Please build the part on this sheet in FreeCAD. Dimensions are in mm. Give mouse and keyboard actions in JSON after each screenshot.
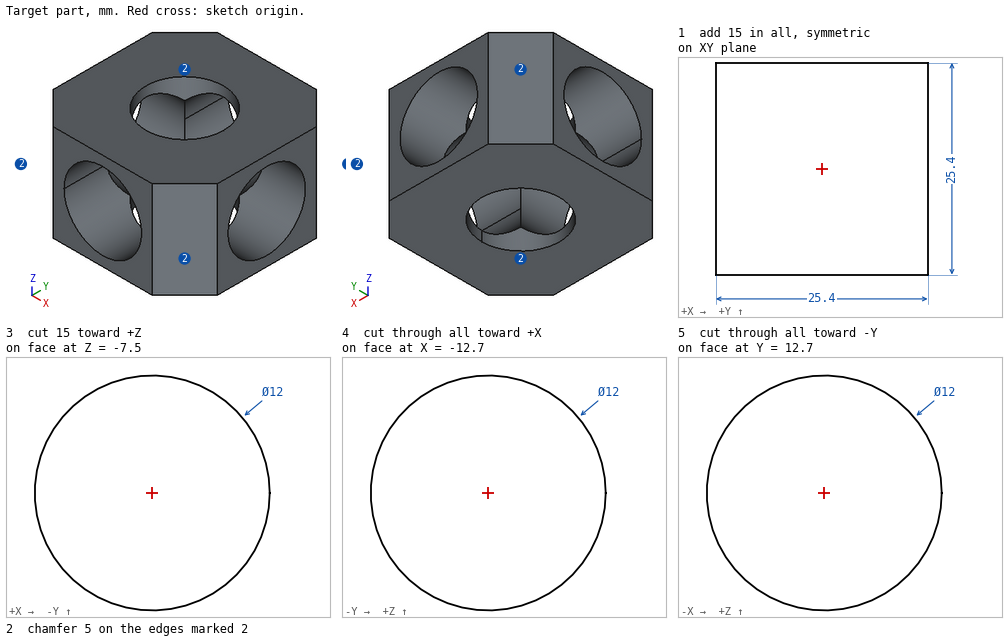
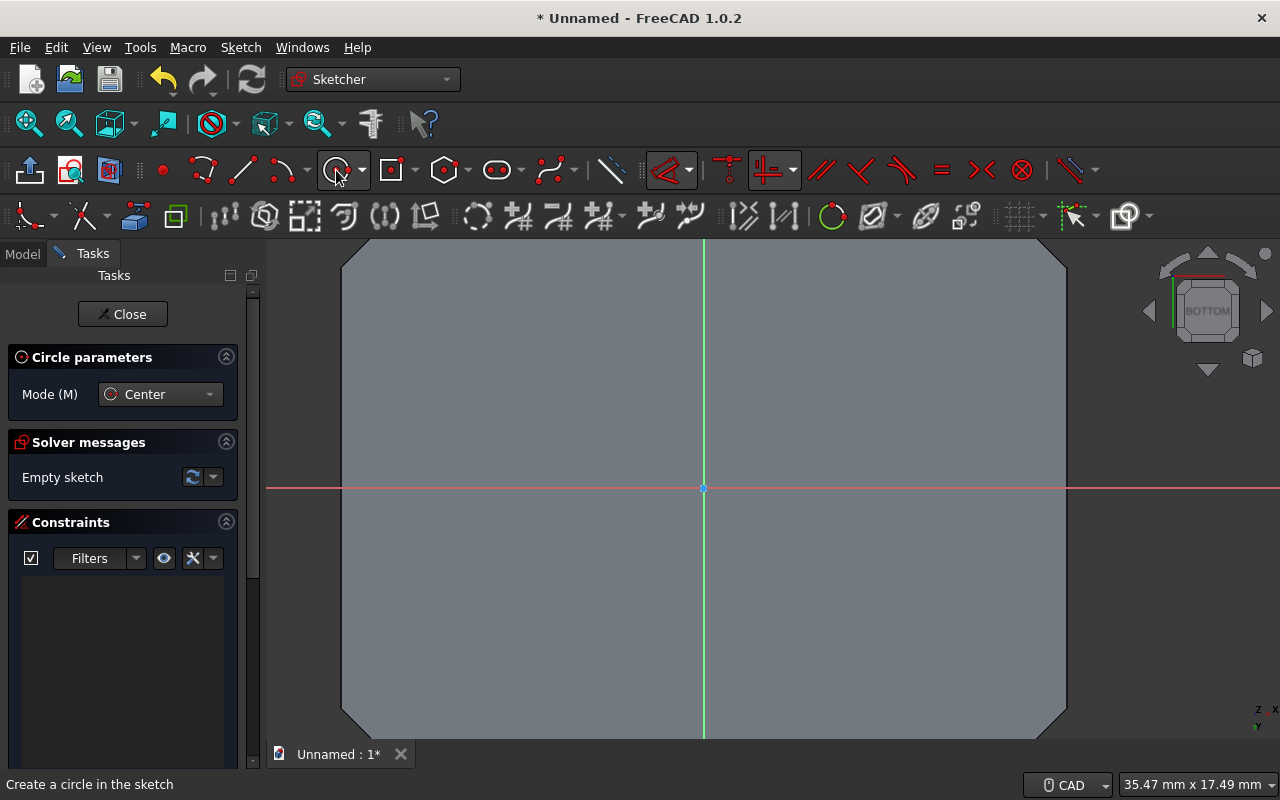
{"action": "left_click", "coordinate": [704, 488]}
{"action": "left_click", "coordinate": [825, 367]}
{"action": "key", "text": "Escape"}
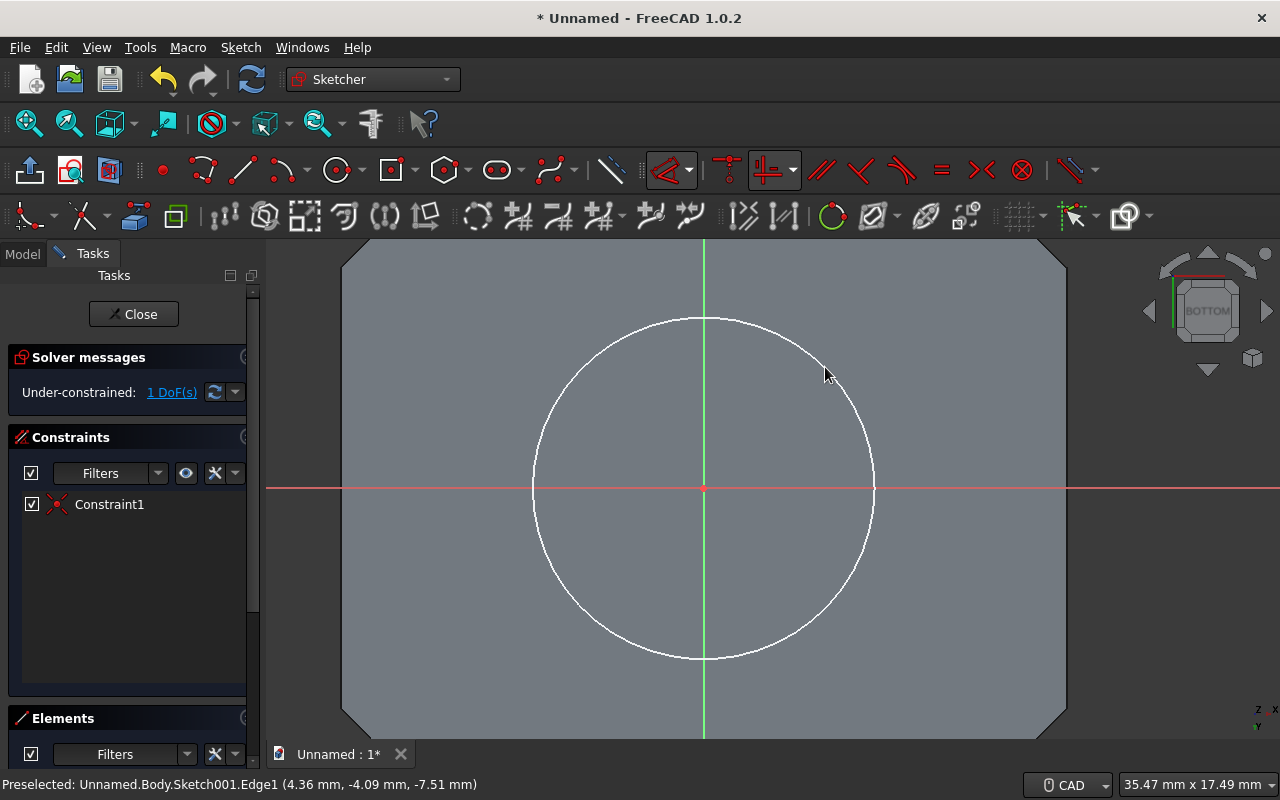
{"action": "left_click", "coordinate": [666, 170]}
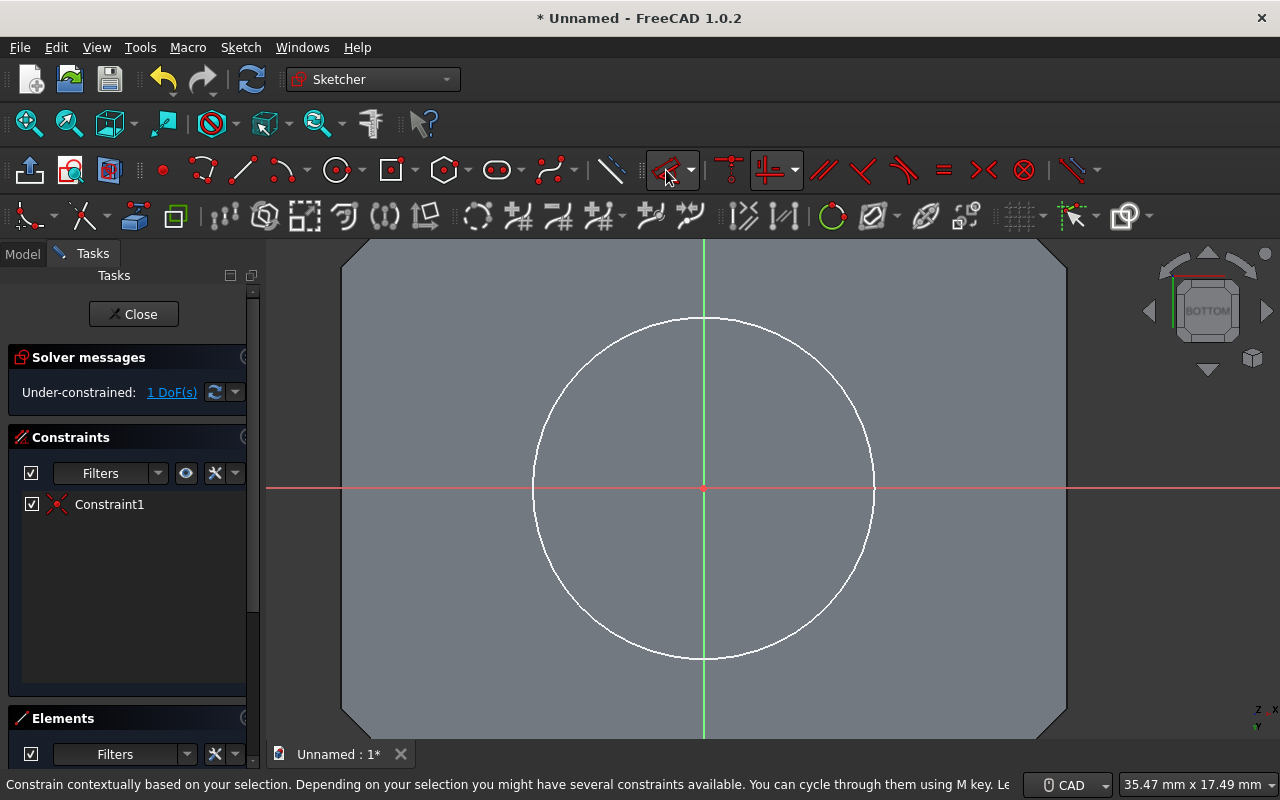
{"action": "left_click", "coordinate": [824, 367]}
{"action": "left_click", "coordinate": [847, 344]}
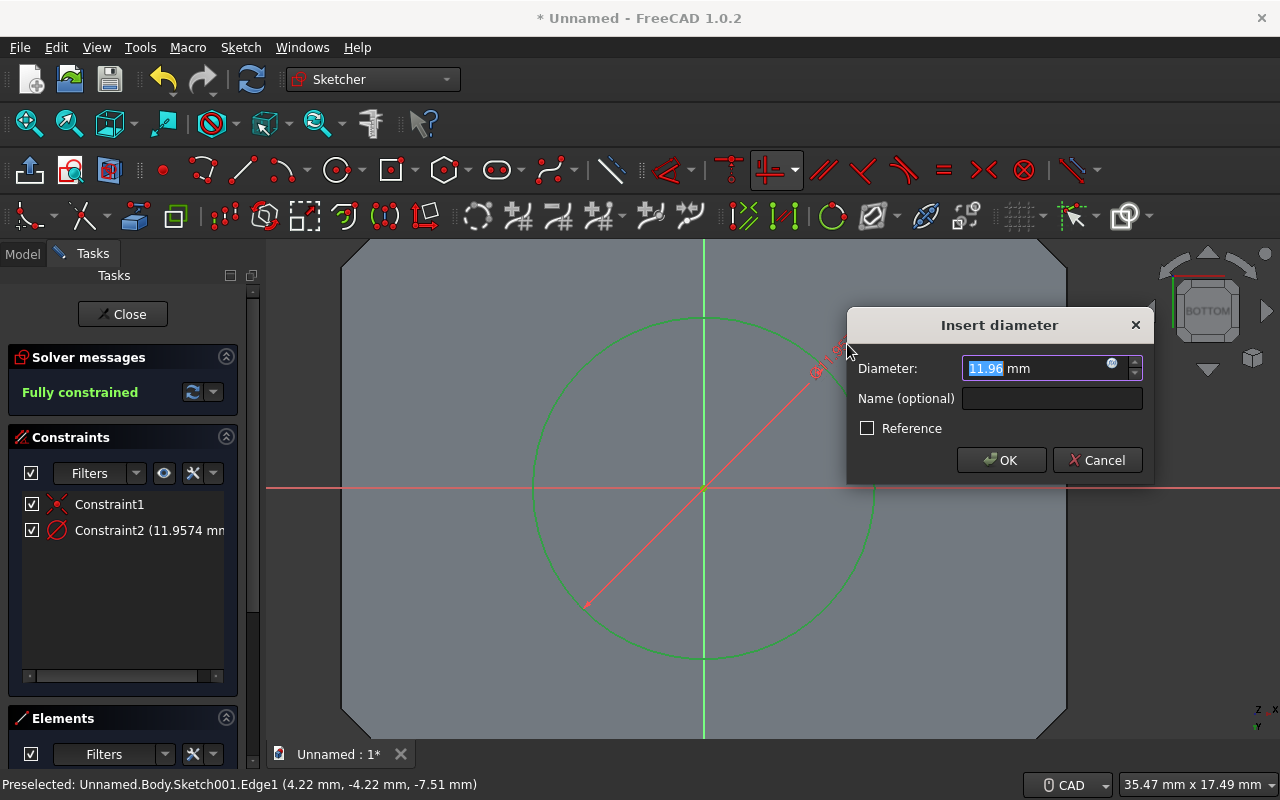
{"action": "type", "text": "12"}
{"action": "key", "text": "Return"}
{"action": "key", "text": "Escape"}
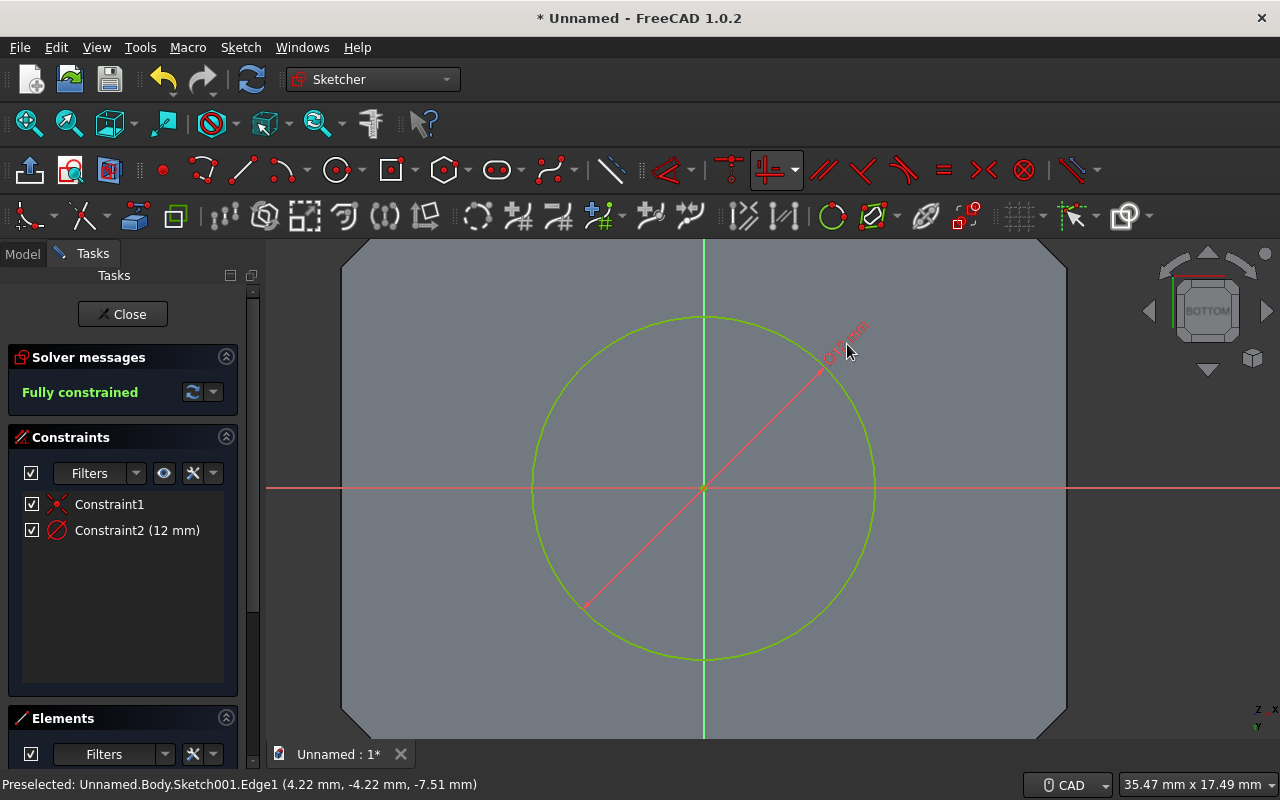
{"action": "left_click", "coordinate": [123, 314]}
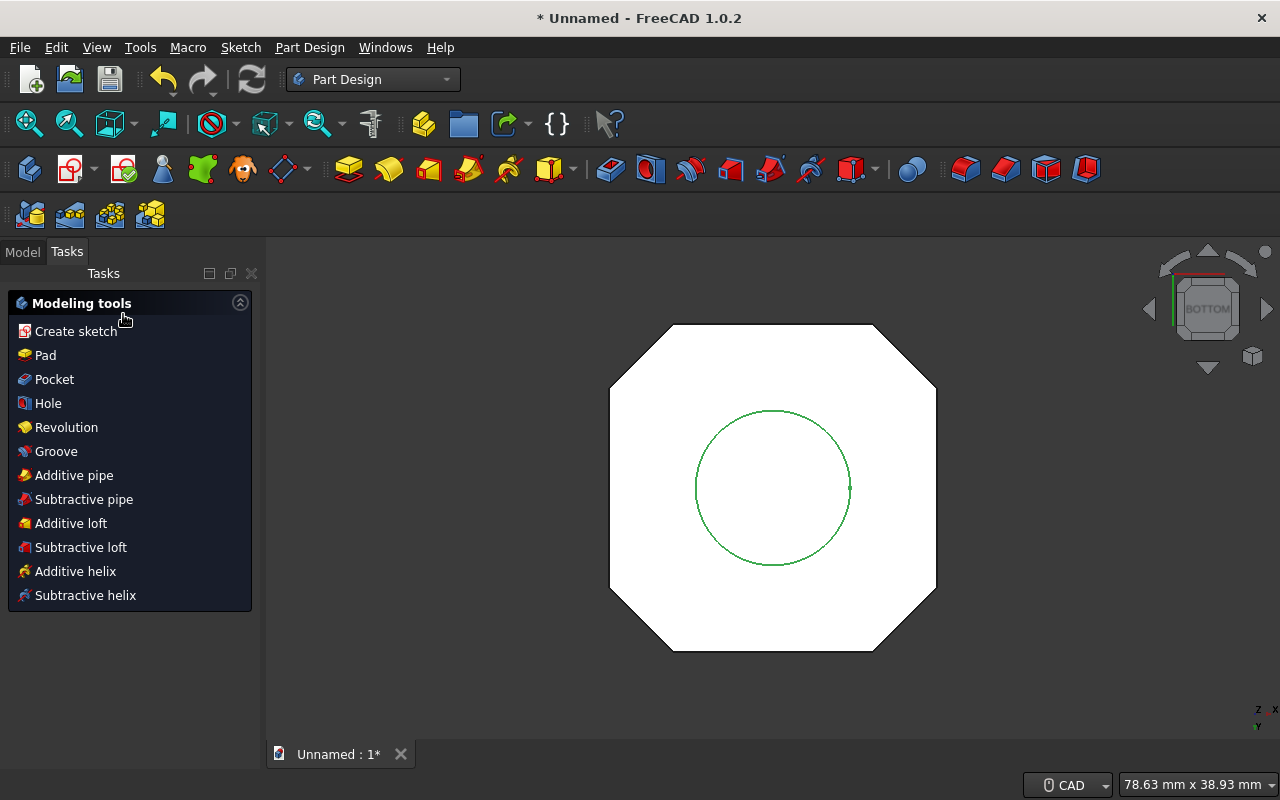
{"action": "left_click", "coordinate": [612, 170]}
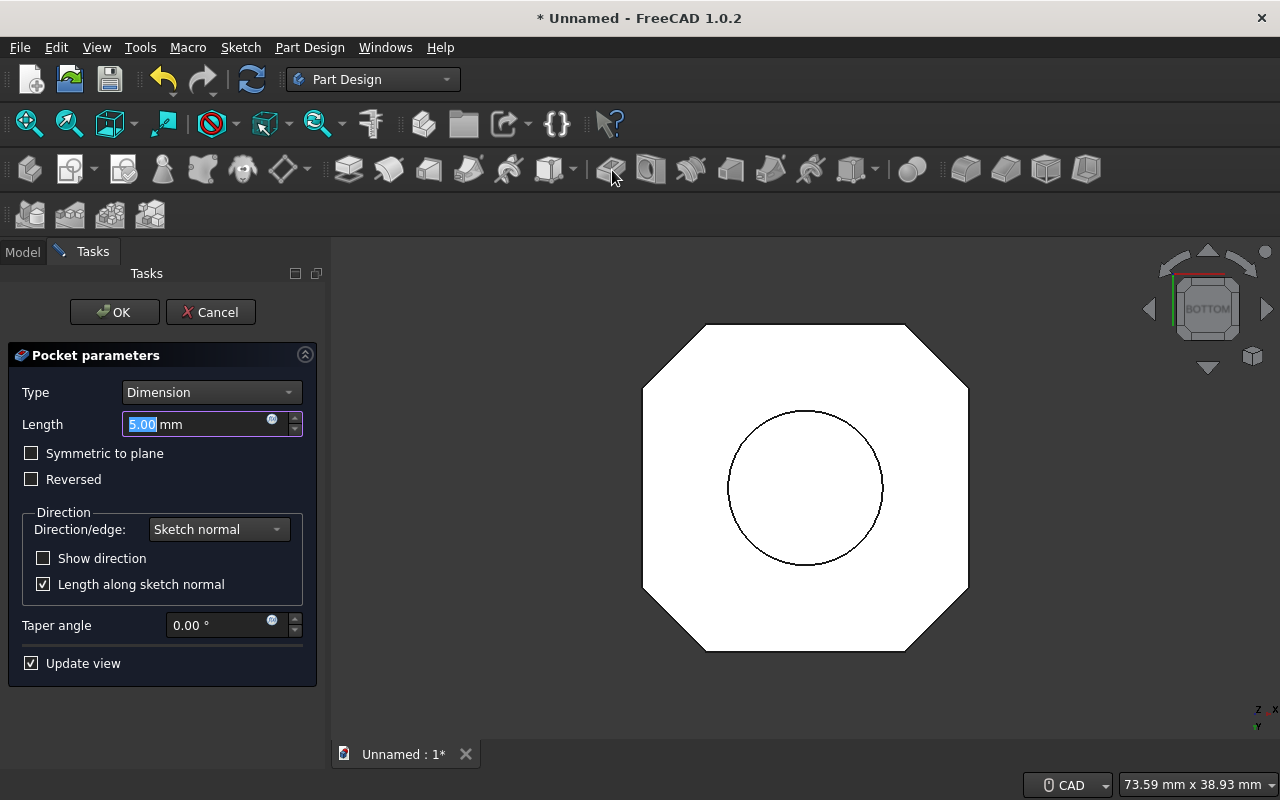
{"action": "type", "text": "15"}
{"action": "key", "text": "Tab"}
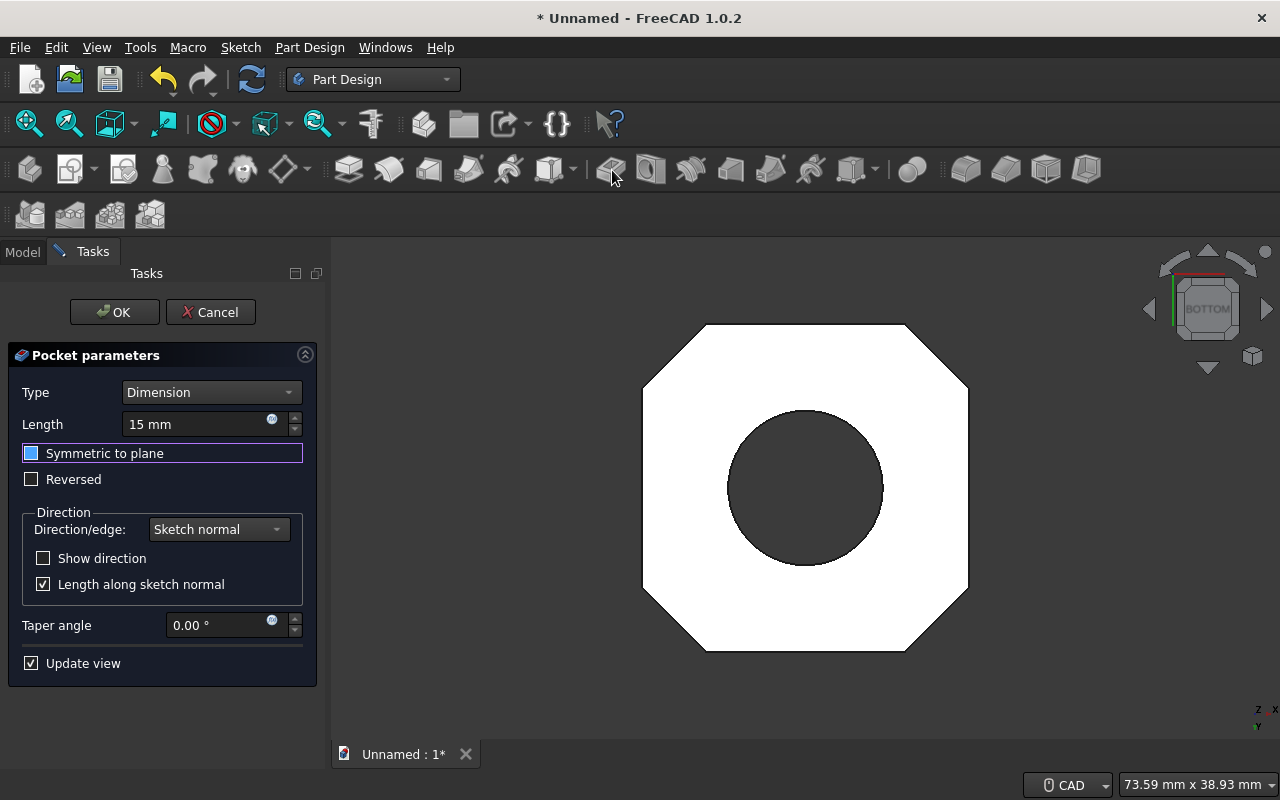
{"action": "left_click", "coordinate": [115, 312]}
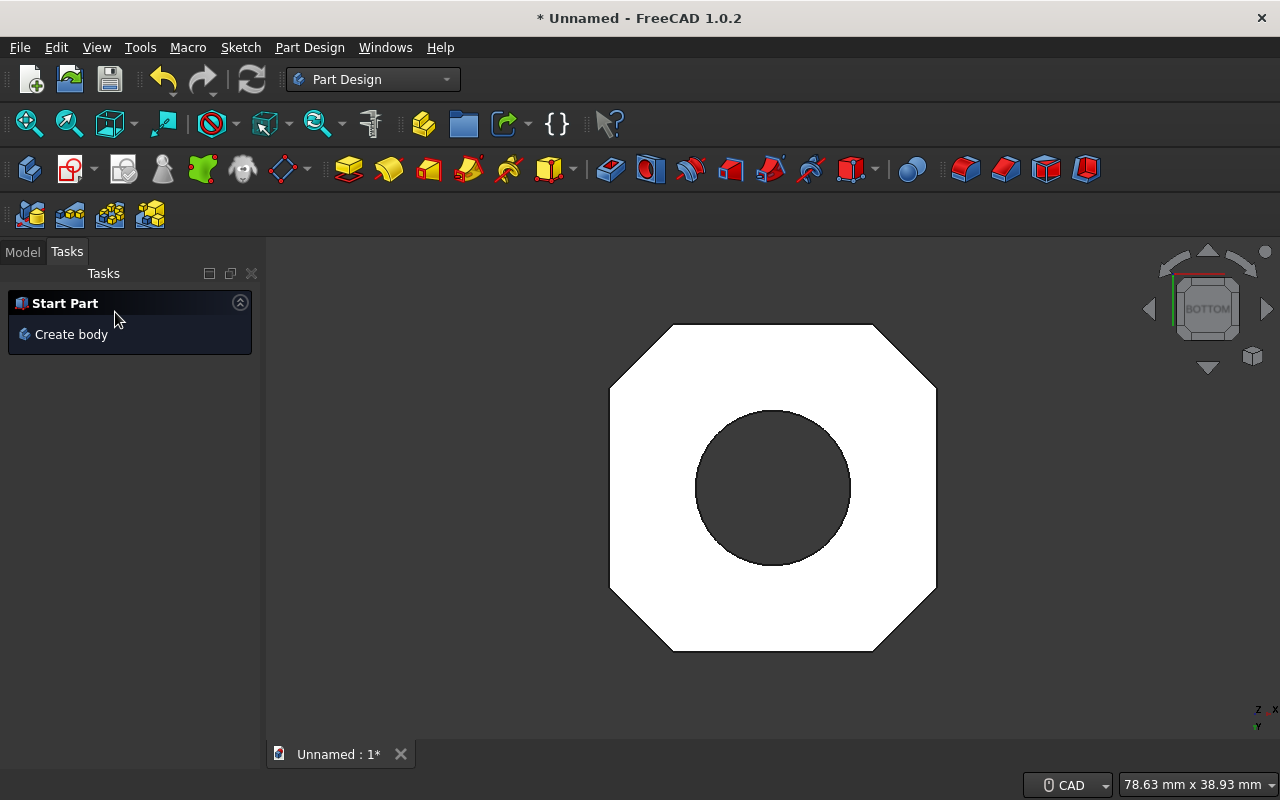
{"action": "key", "text": "6"}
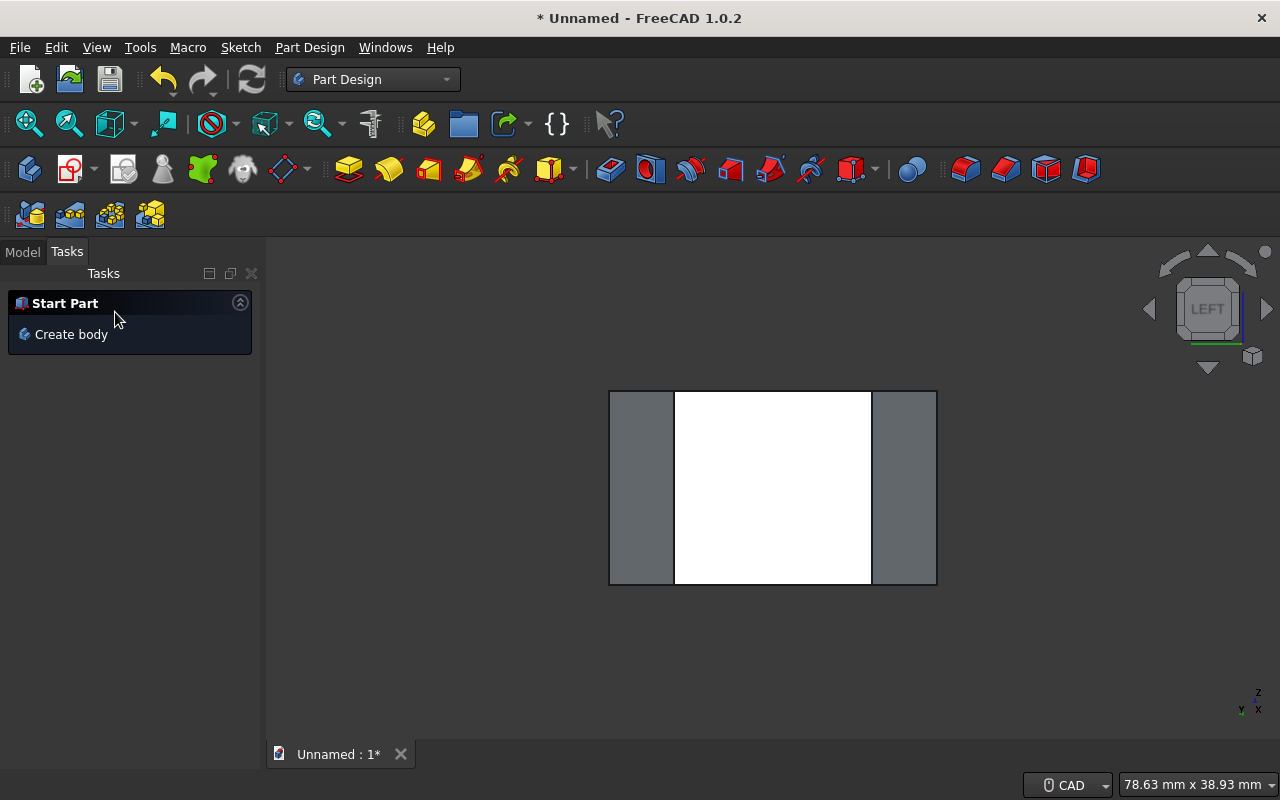
{"action": "key", "text": "v f"}